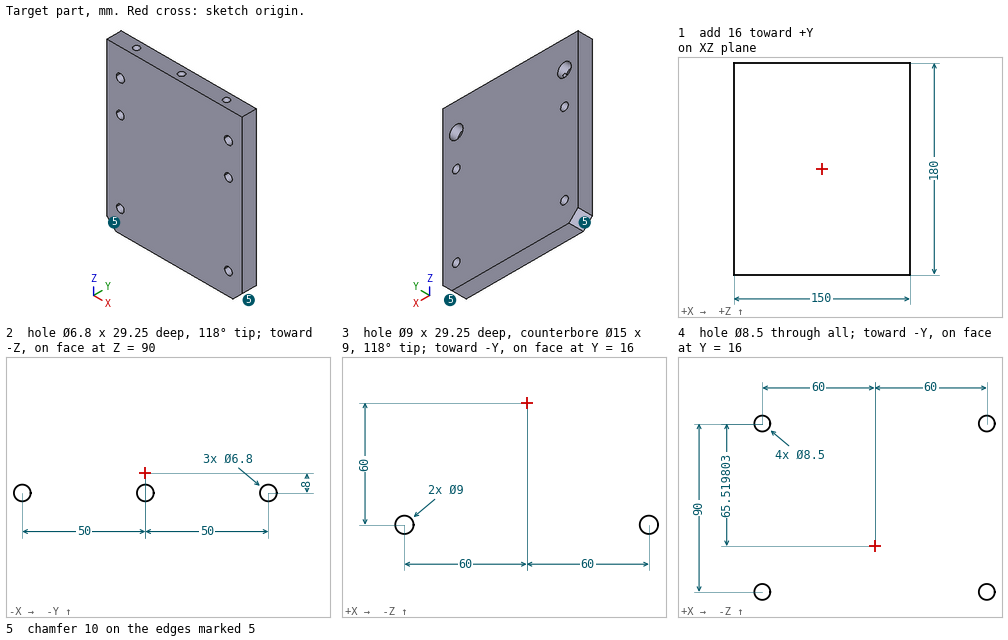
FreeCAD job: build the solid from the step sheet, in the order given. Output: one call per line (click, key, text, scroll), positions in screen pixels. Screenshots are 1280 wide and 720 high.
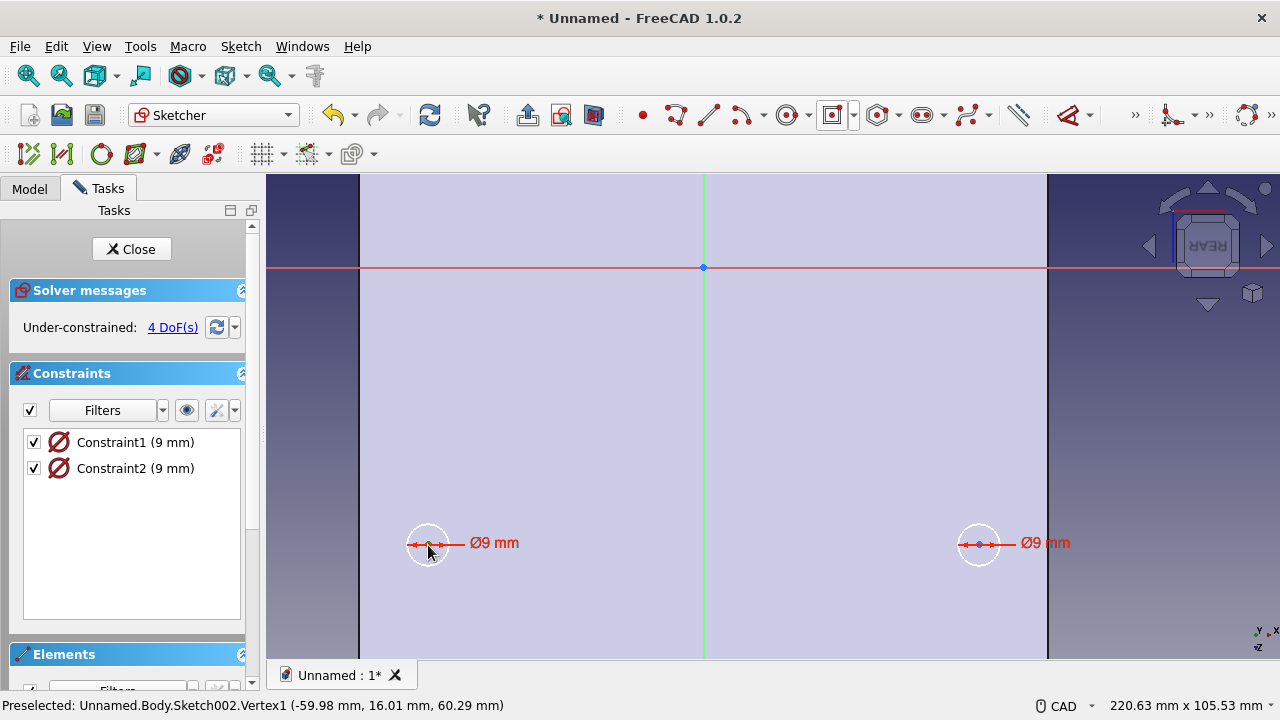
click(979, 545)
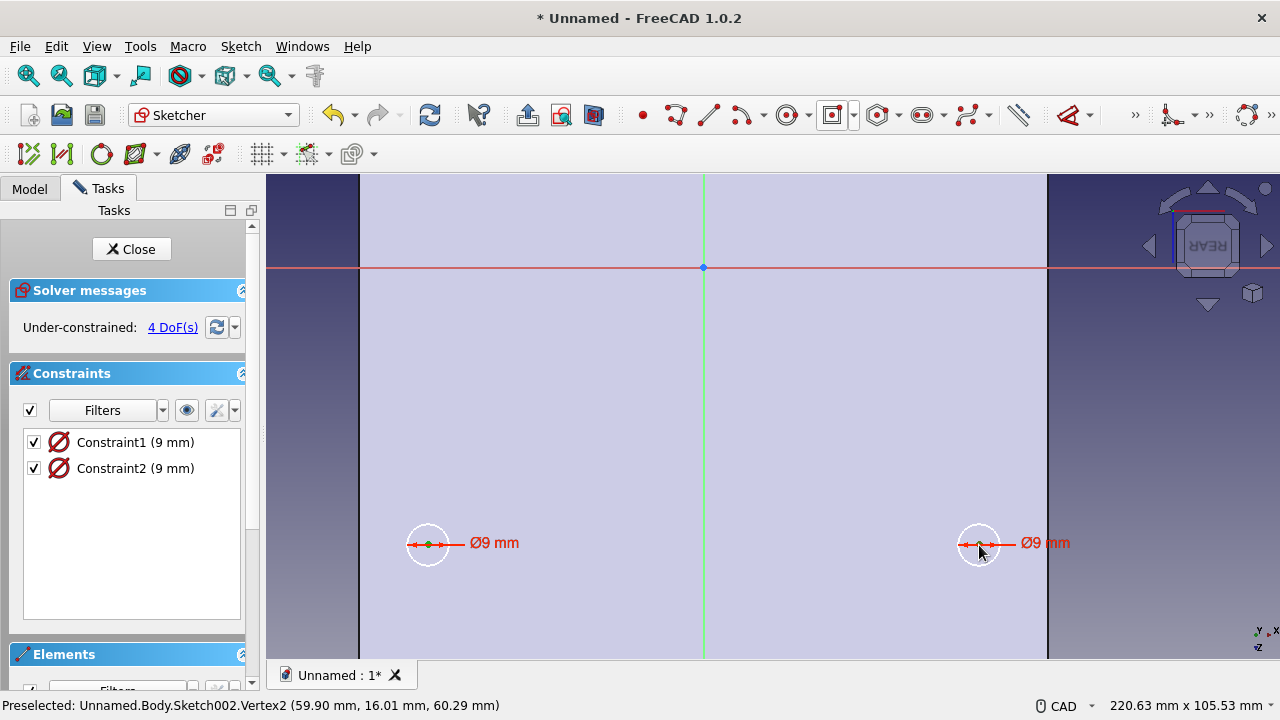
key(h)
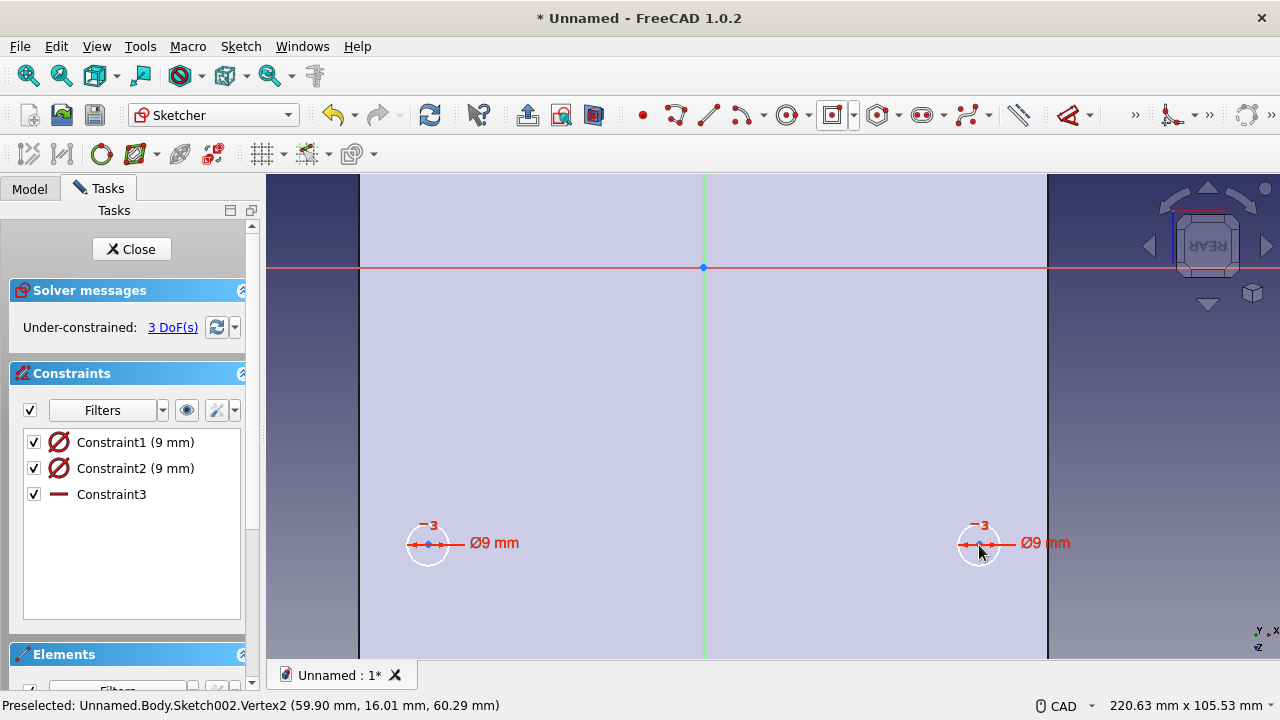
click(1068, 116)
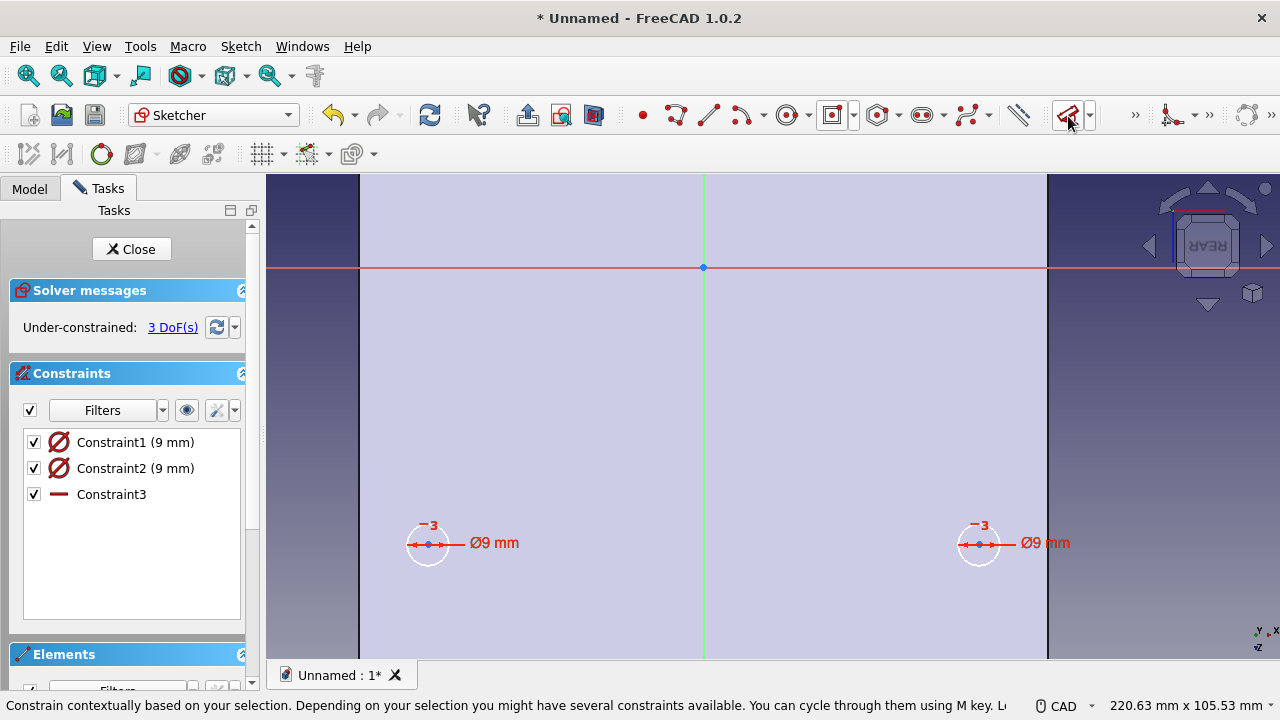
click(428, 545)
click(566, 234)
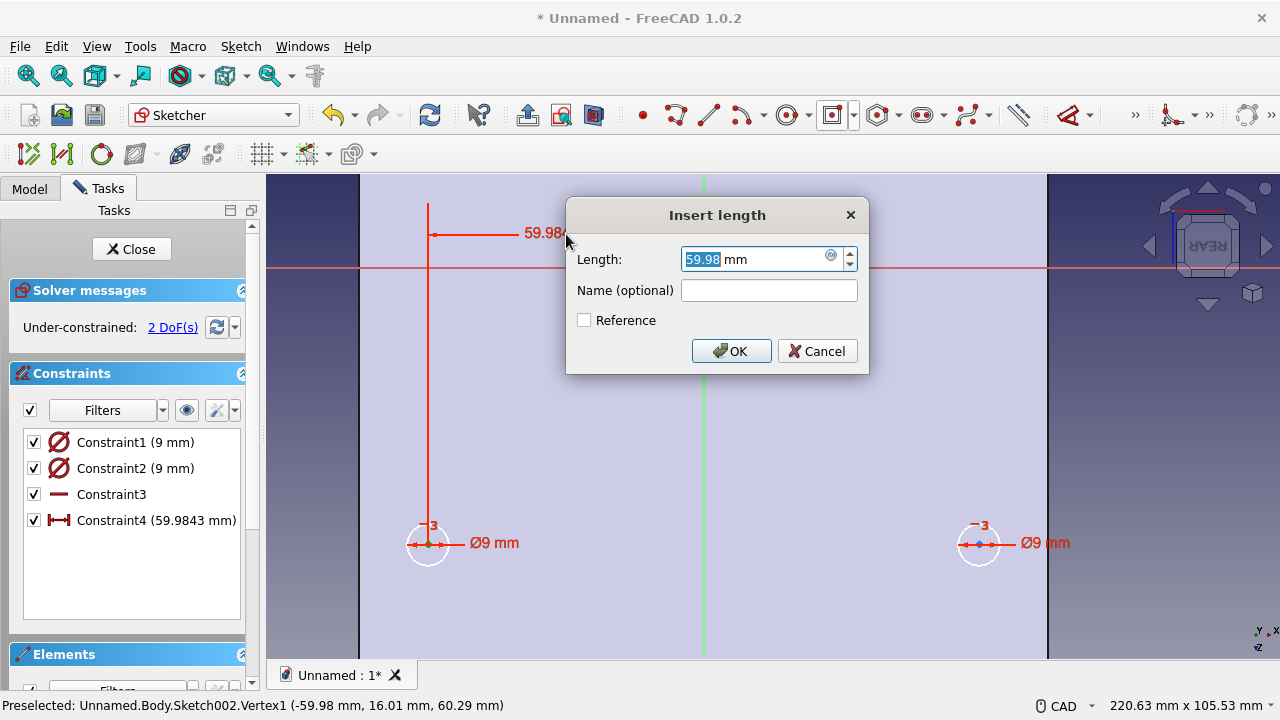
text(60)
key(Return)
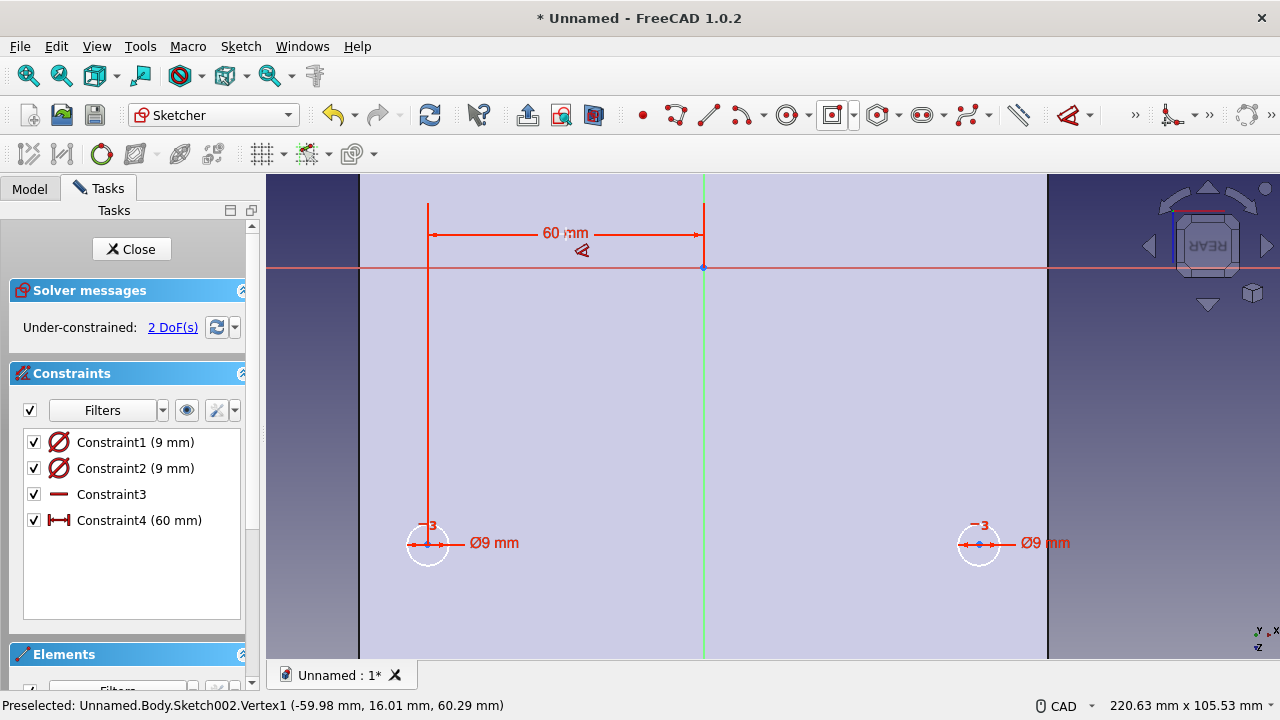
click(428, 545)
click(394, 406)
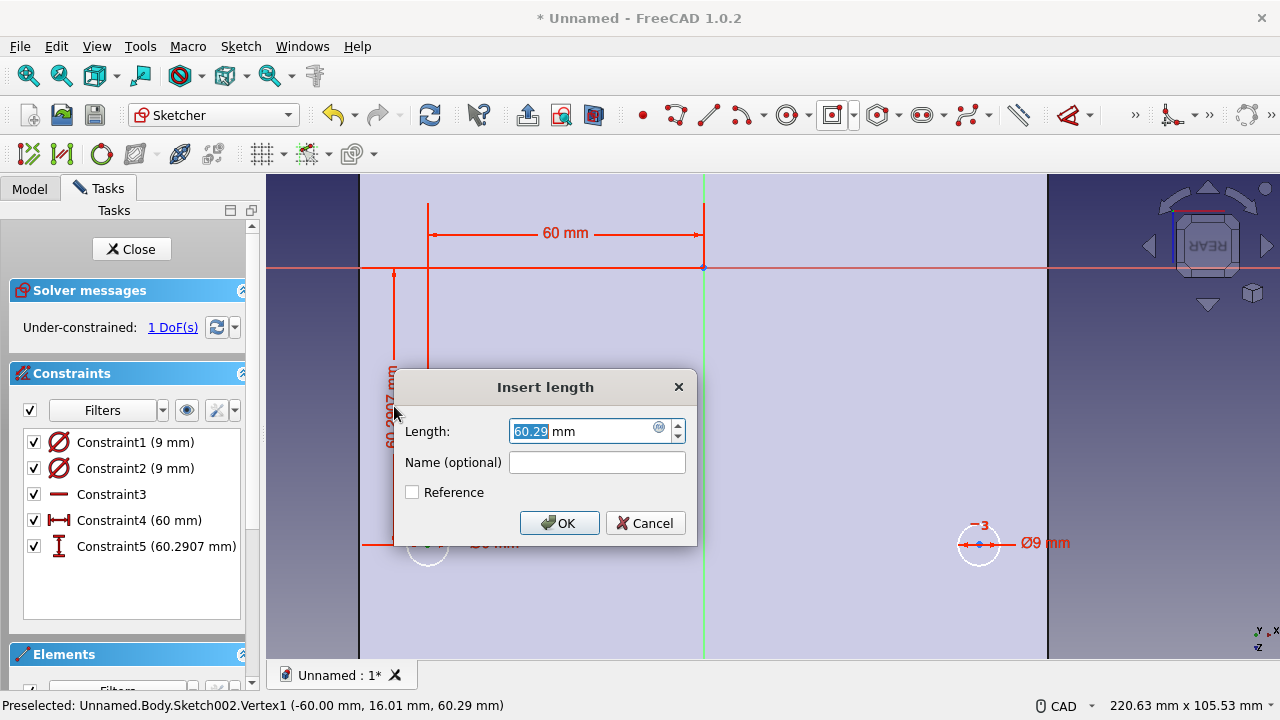
text(60)
key(Return)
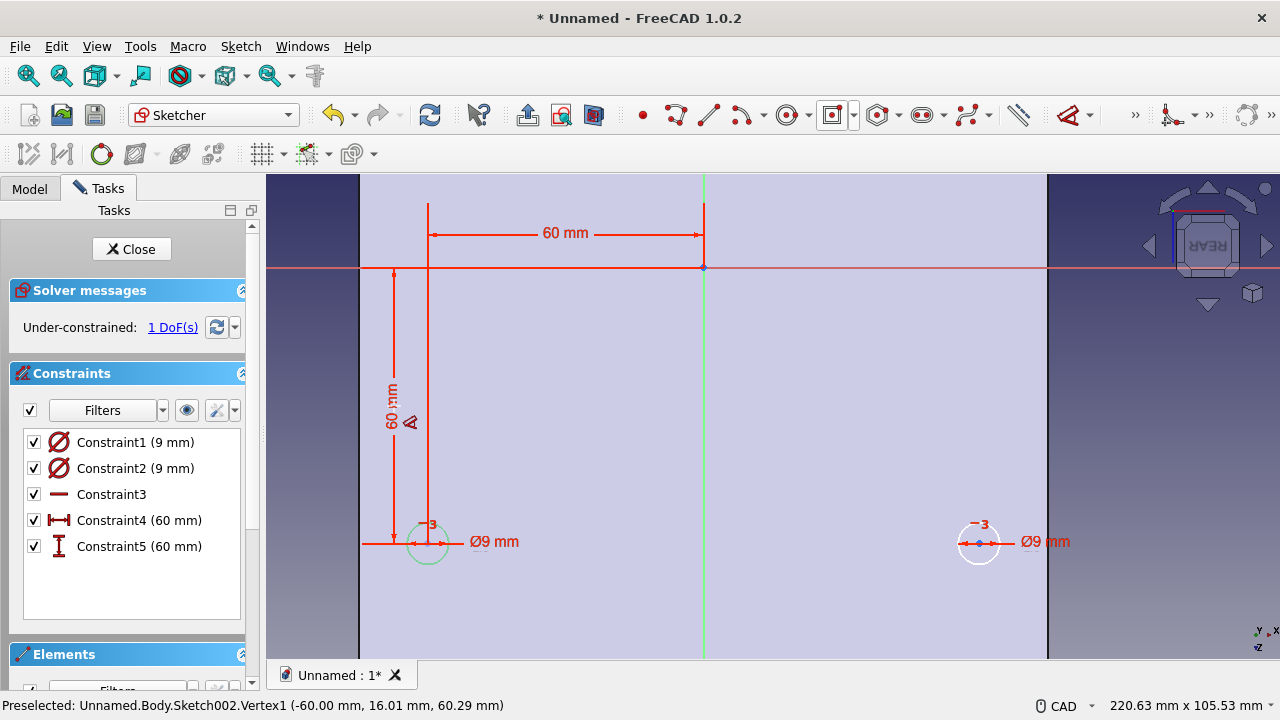
click(979, 544)
click(841, 234)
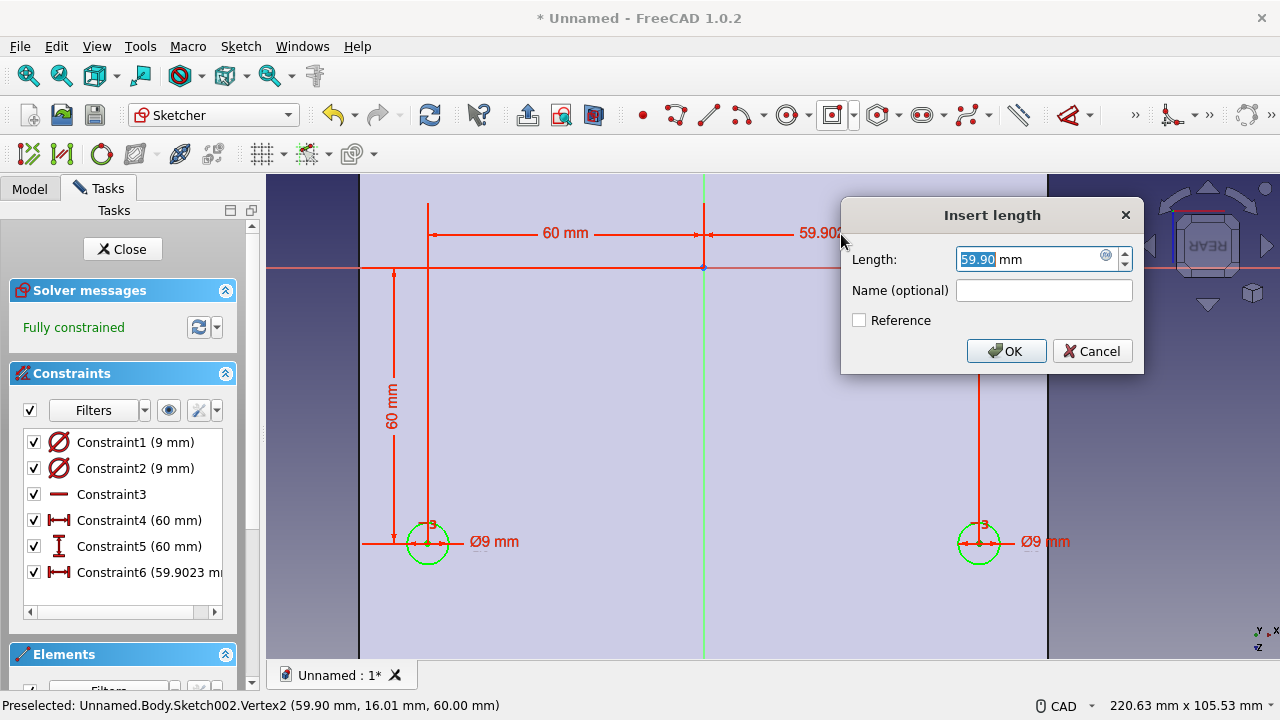
text(60)
key(Return)
key(Escape)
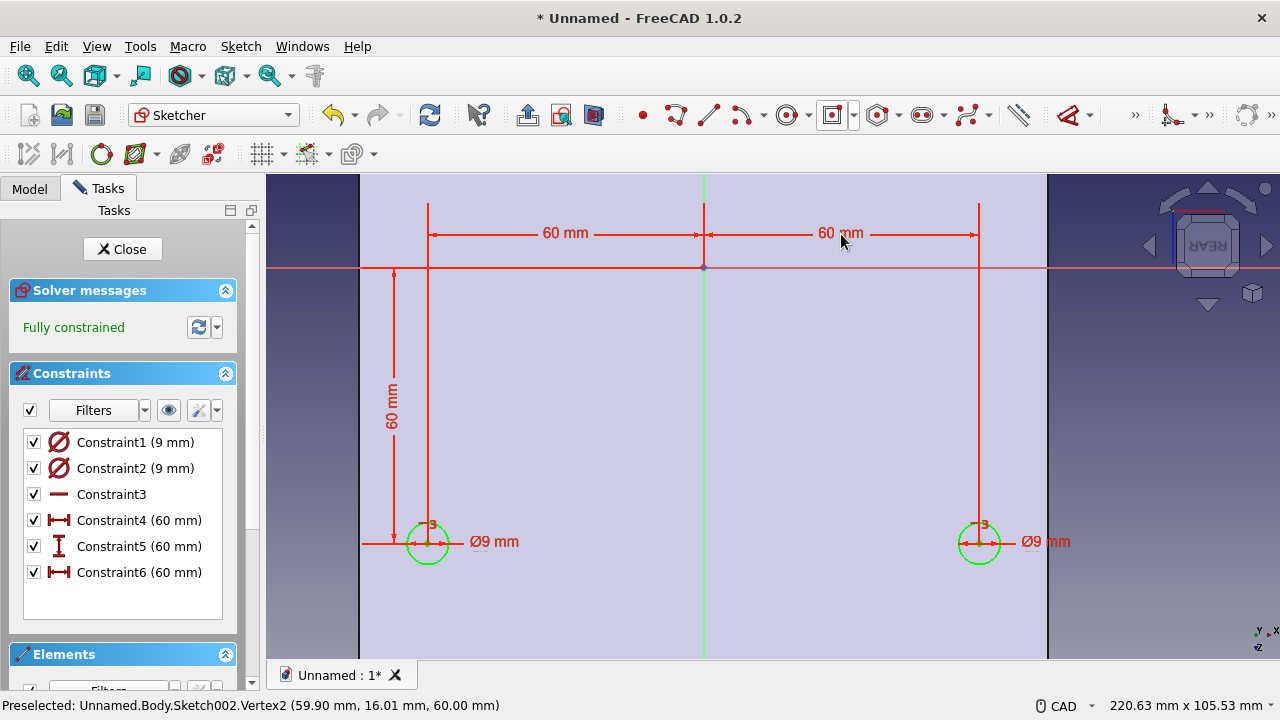
click(123, 249)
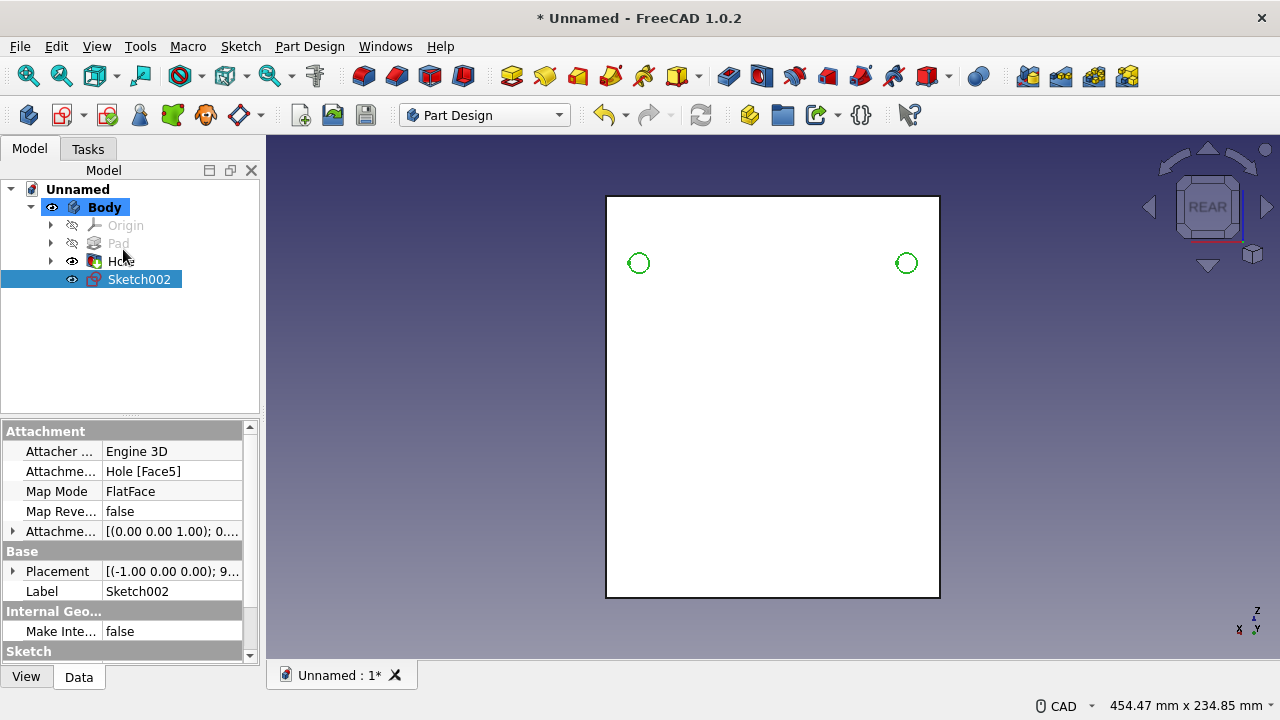
click(762, 76)